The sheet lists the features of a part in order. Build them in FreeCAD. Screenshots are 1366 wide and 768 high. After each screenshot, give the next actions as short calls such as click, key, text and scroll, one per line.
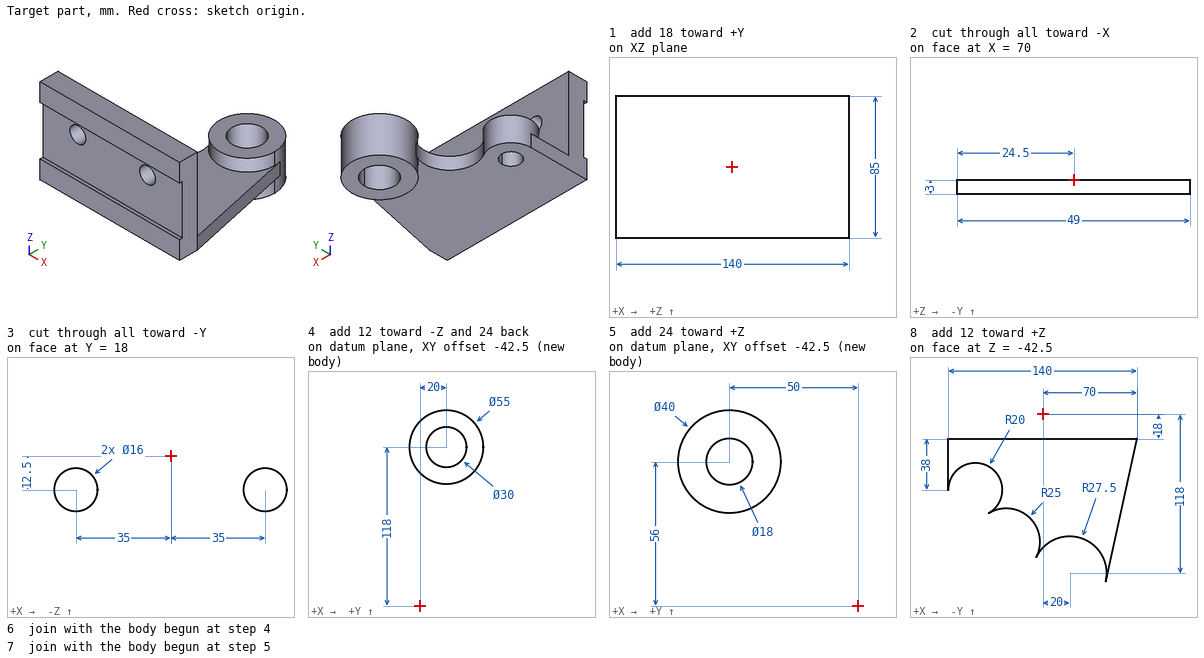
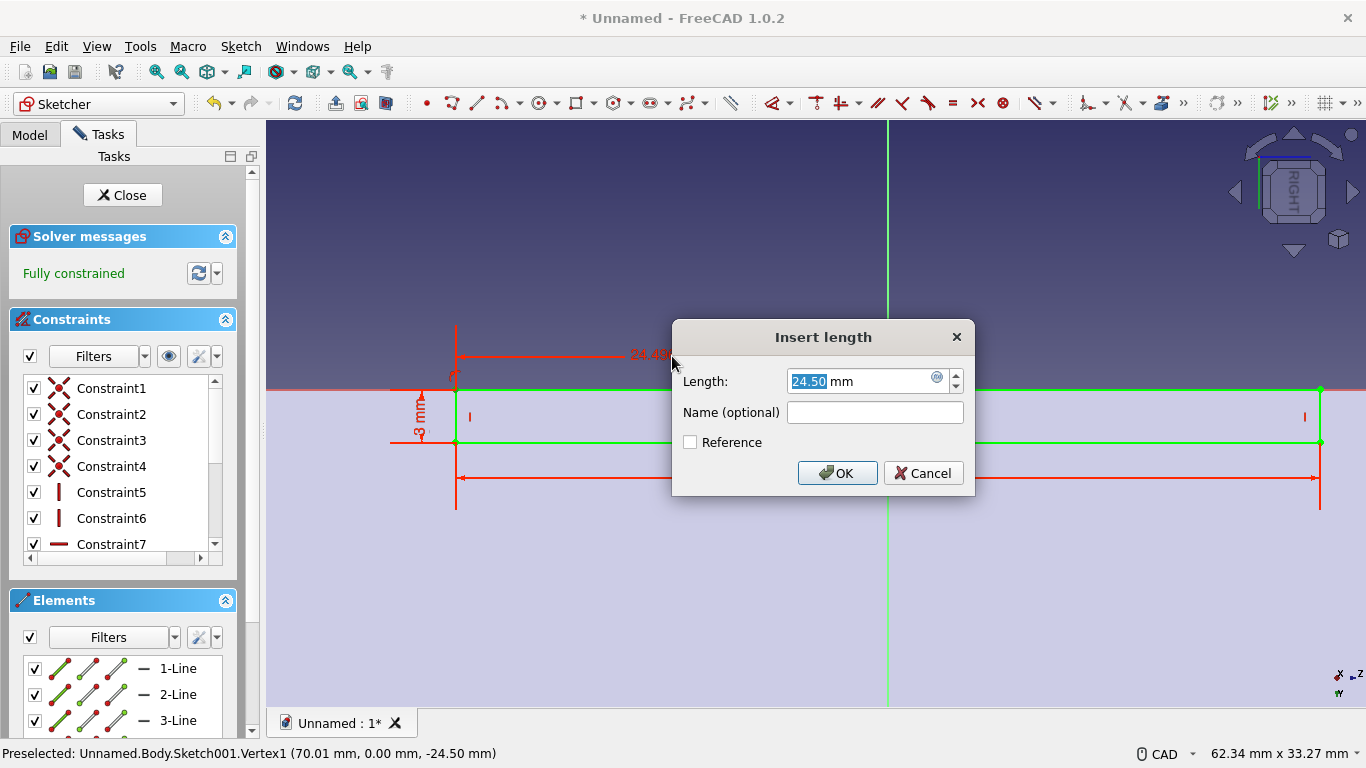
text(24.5)
key(Return)
key(Escape)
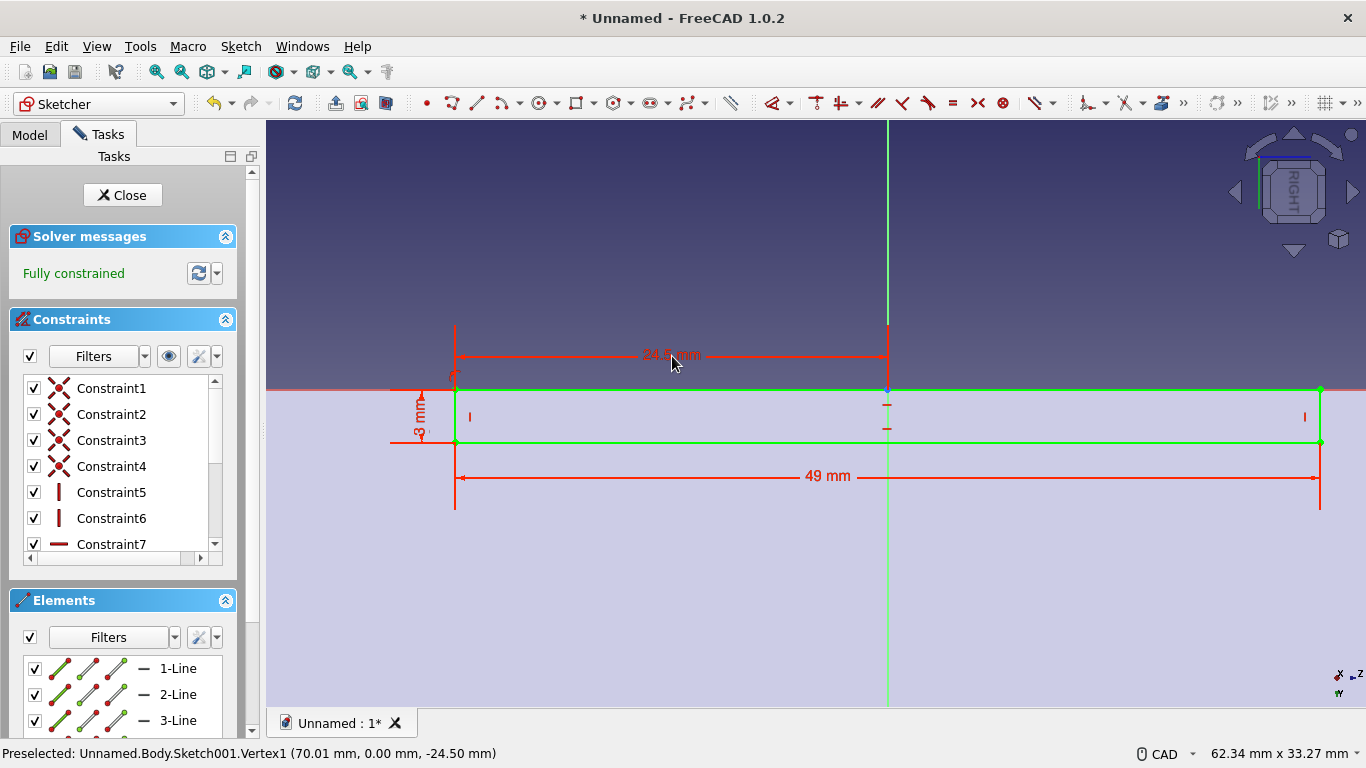
click(123, 195)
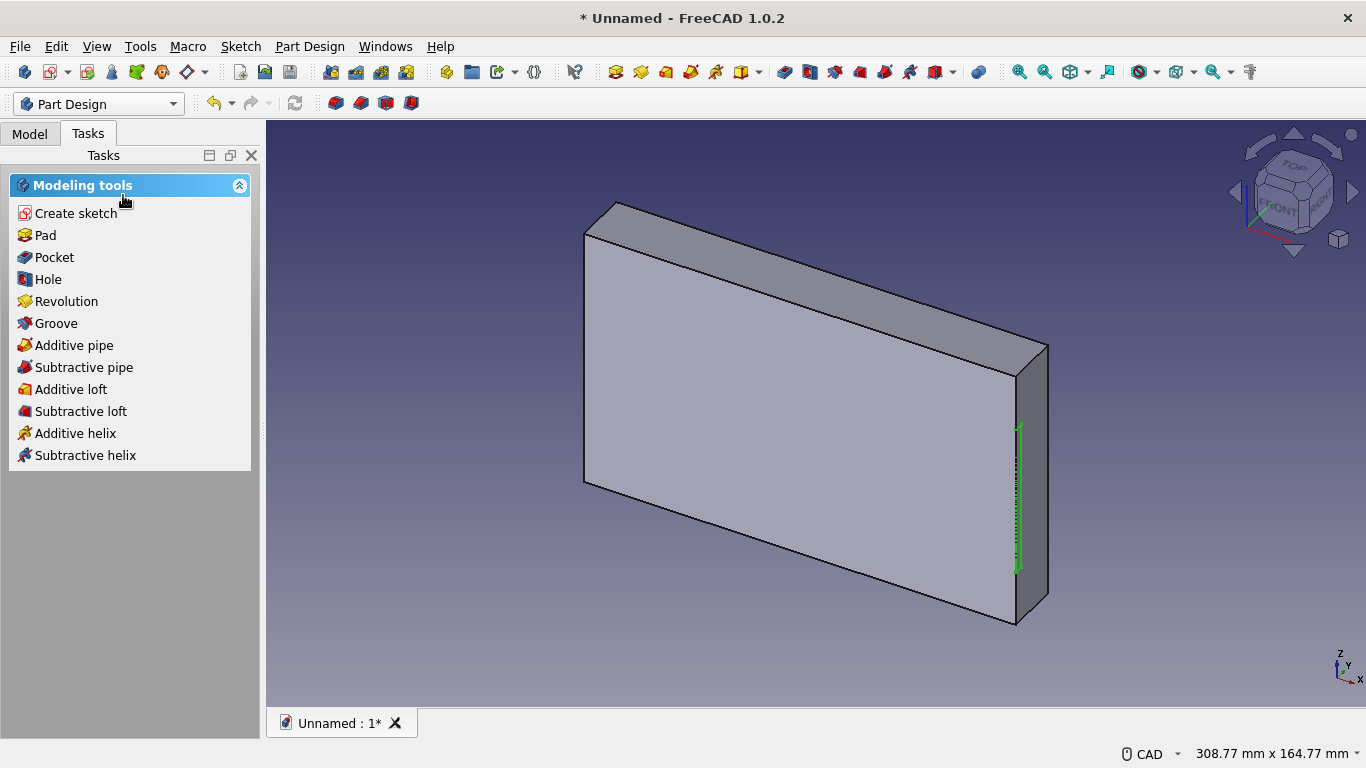
click(785, 72)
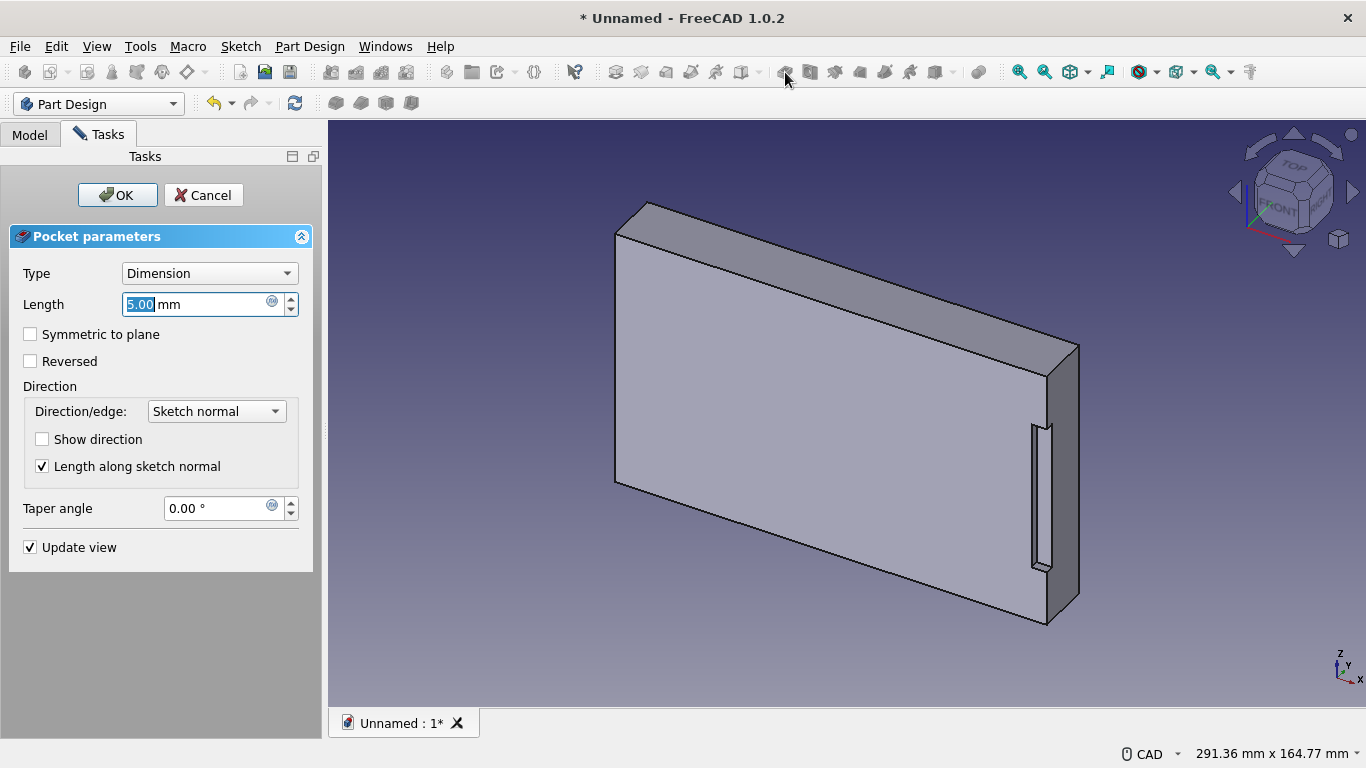
click(210, 274)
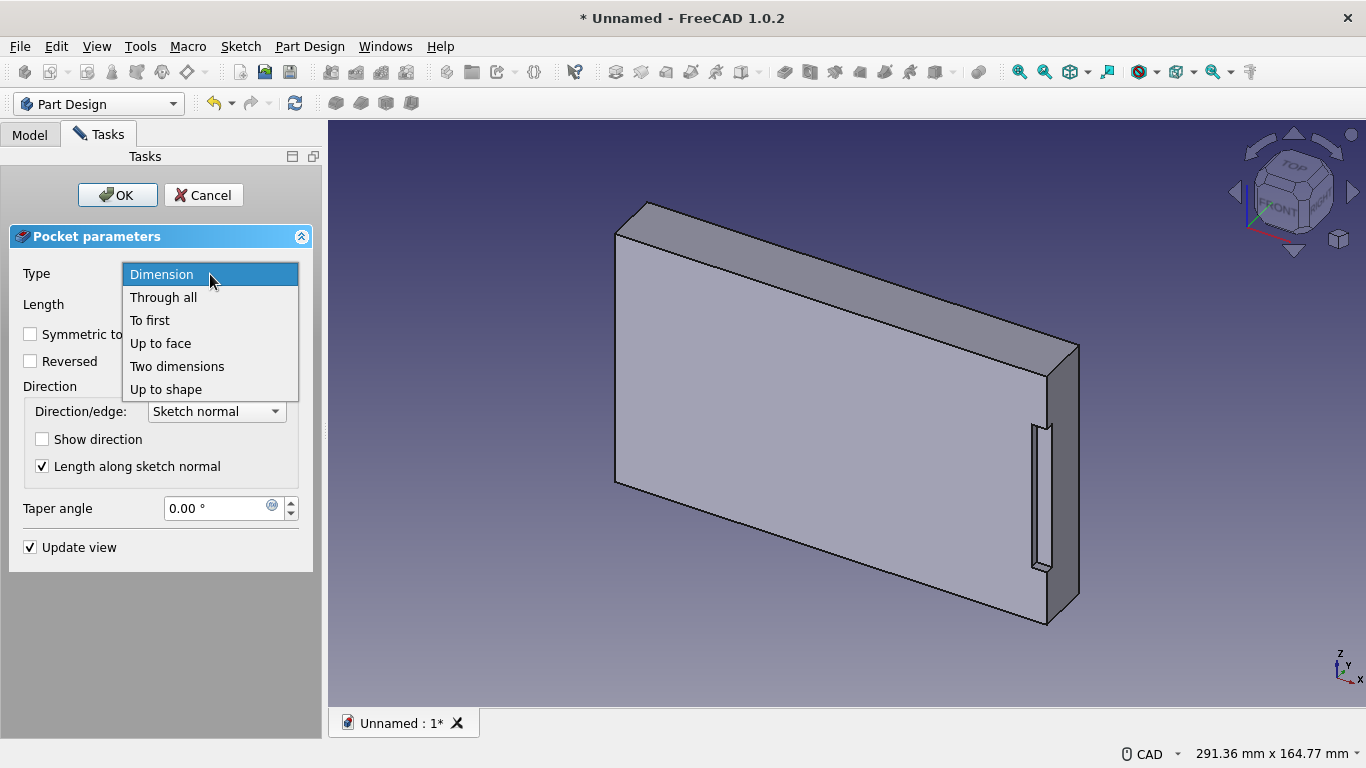
click(208, 298)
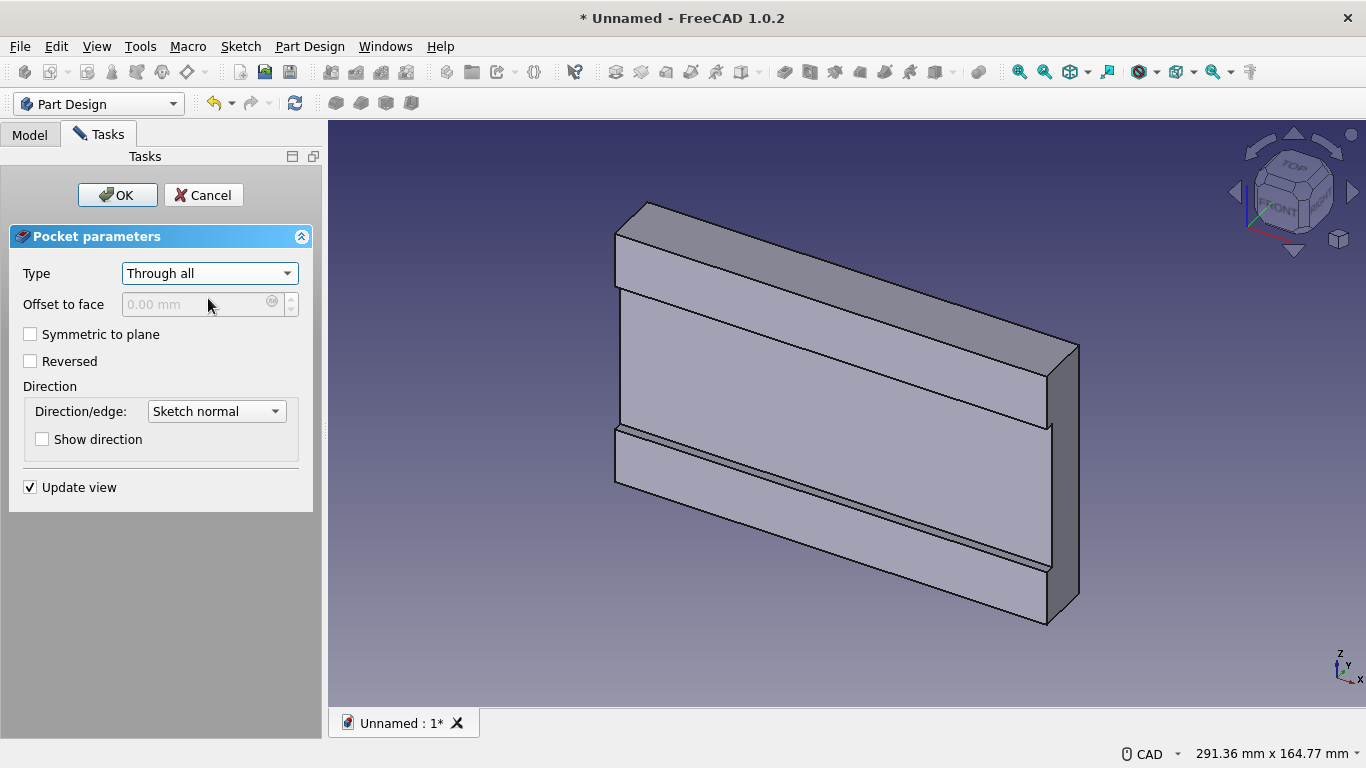
click(118, 195)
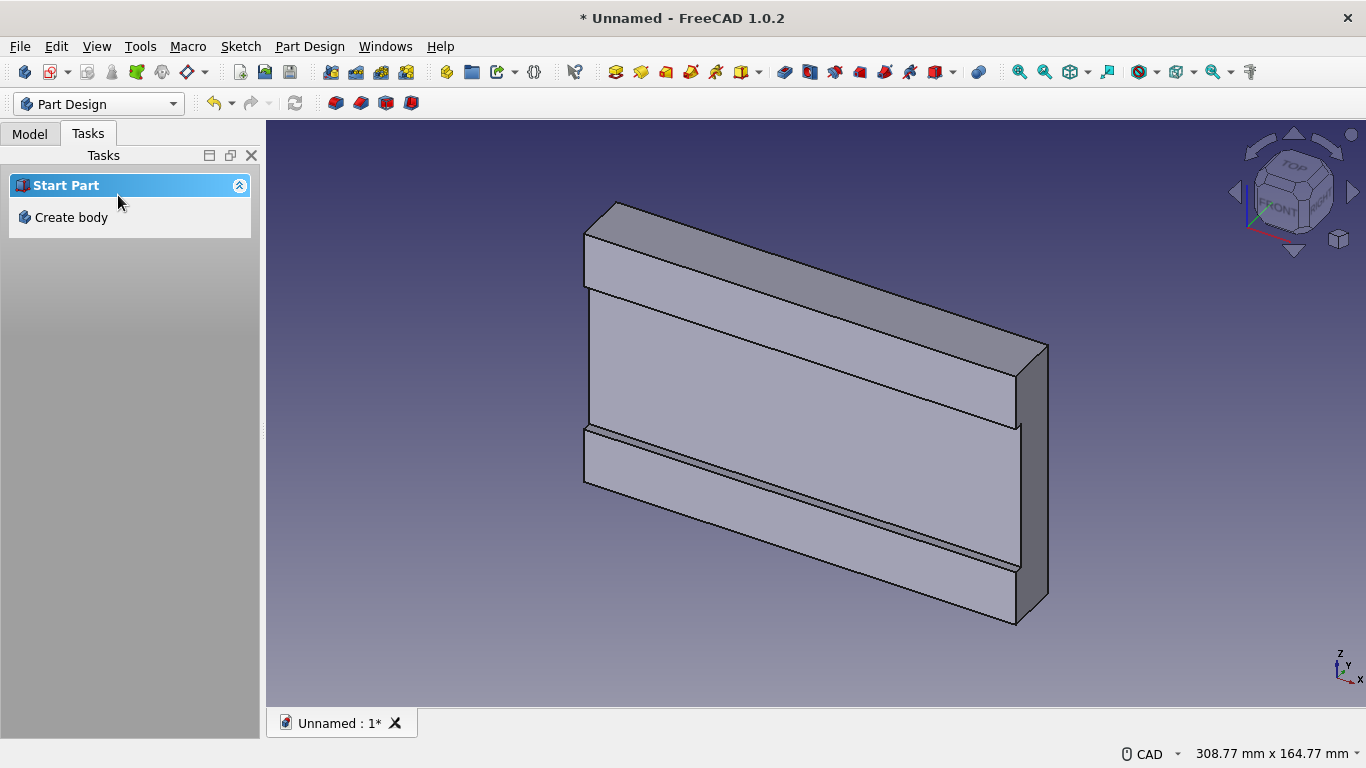
key(4)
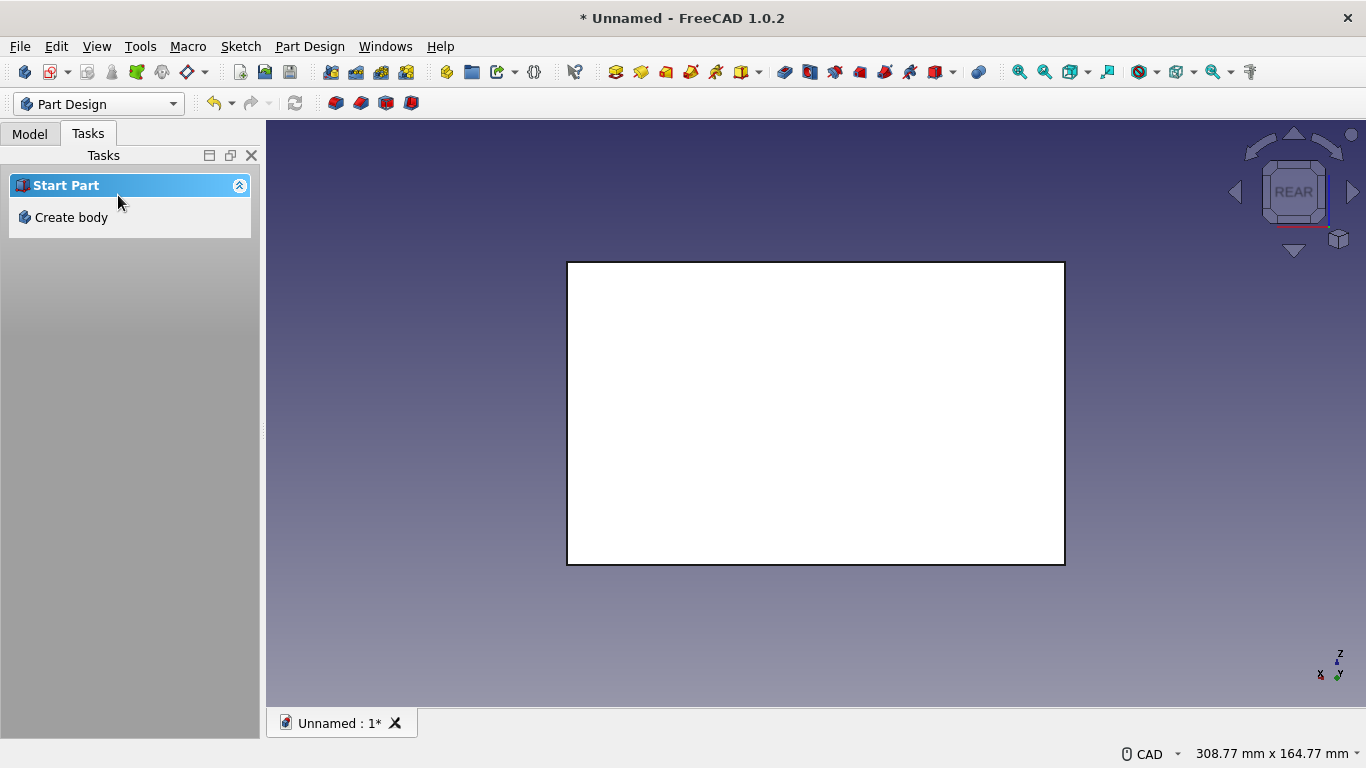
click(745, 413)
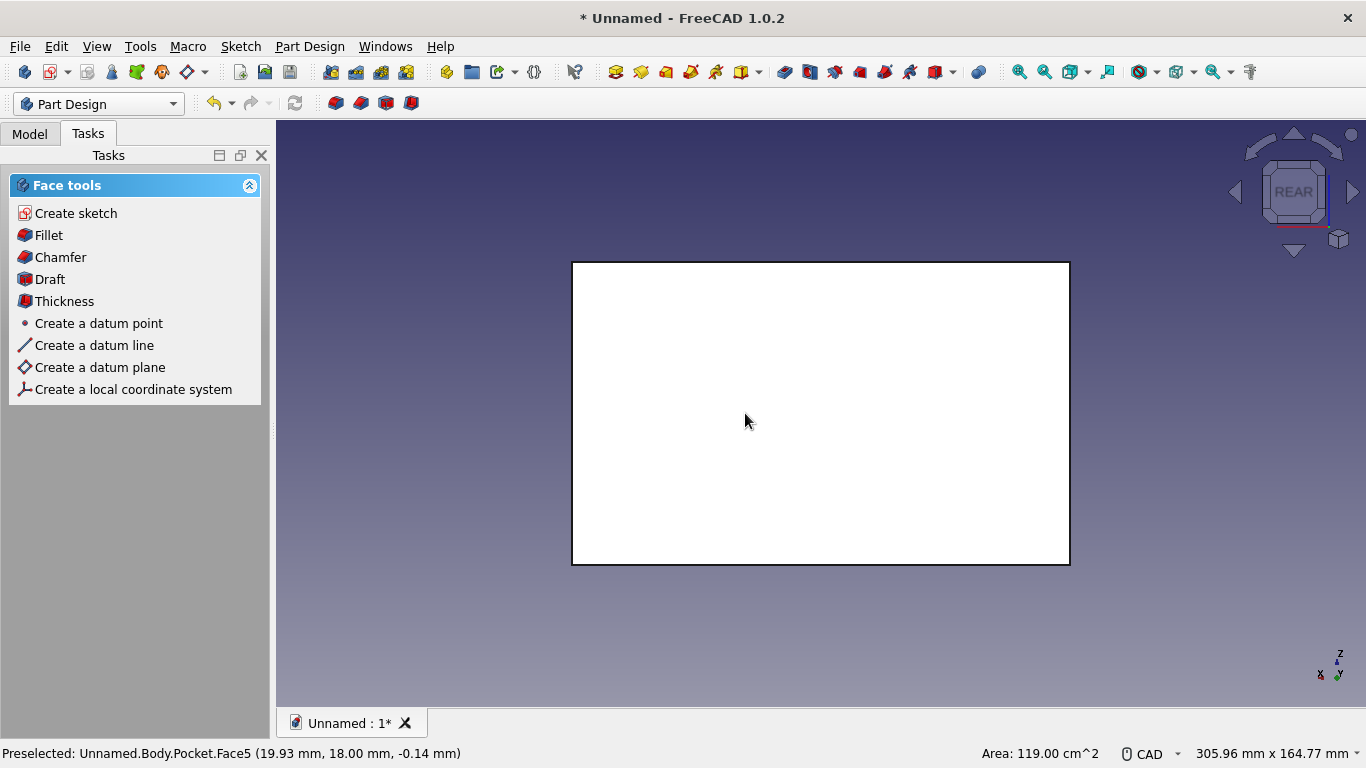
click(50, 72)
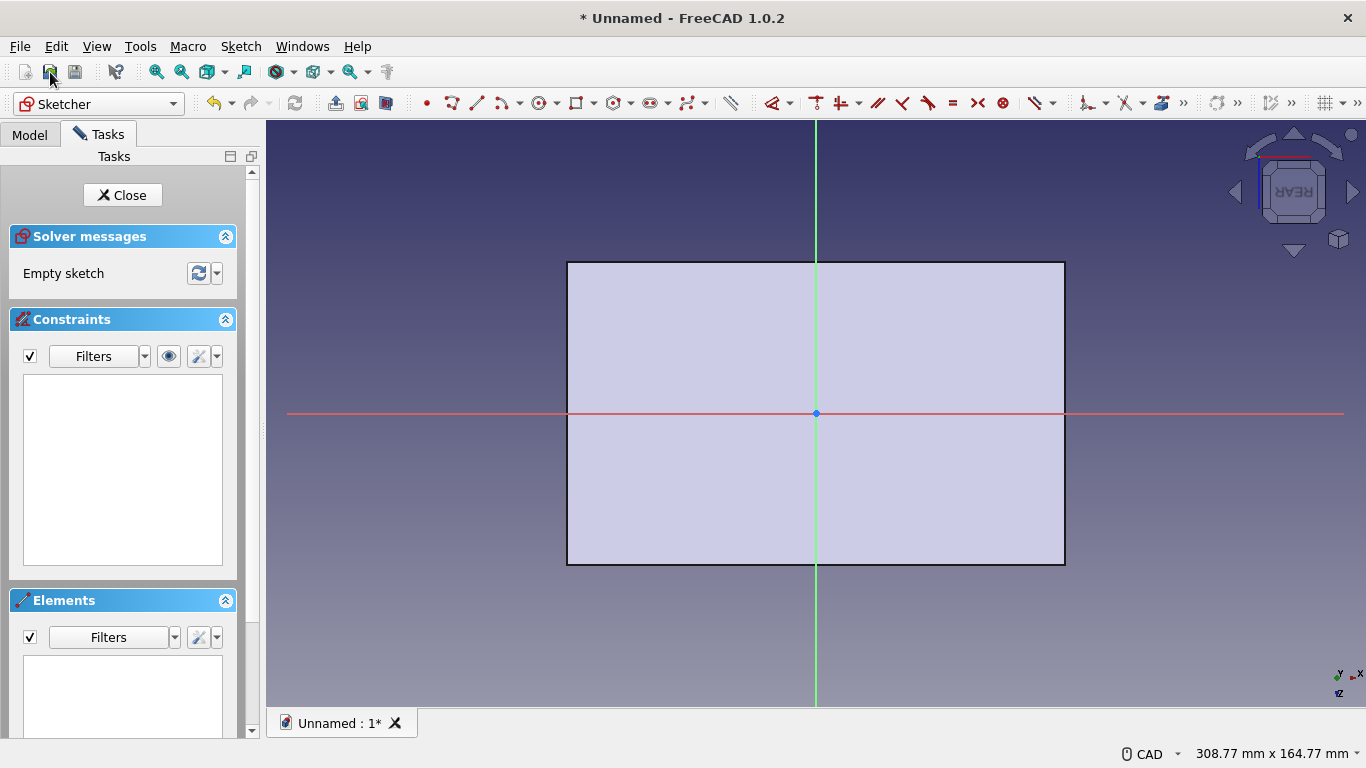
scroll(872, 480, up, 4)